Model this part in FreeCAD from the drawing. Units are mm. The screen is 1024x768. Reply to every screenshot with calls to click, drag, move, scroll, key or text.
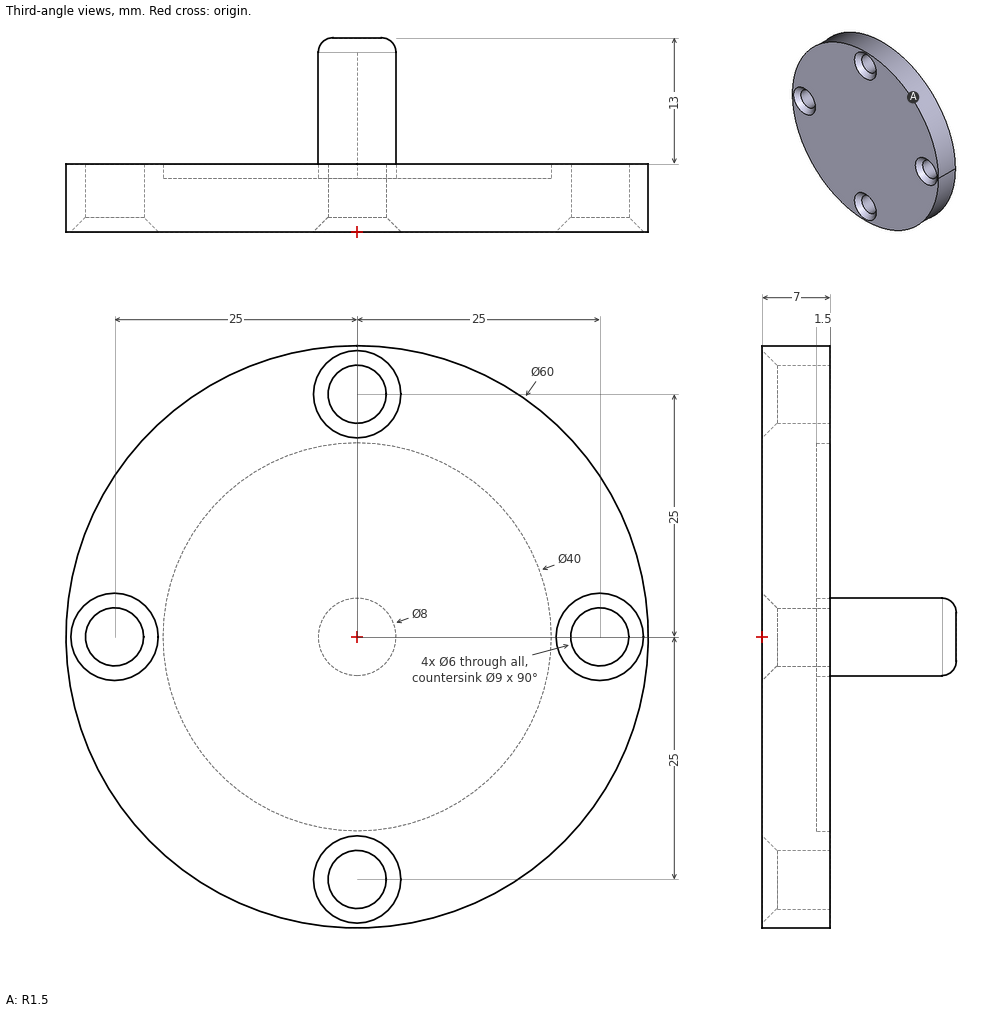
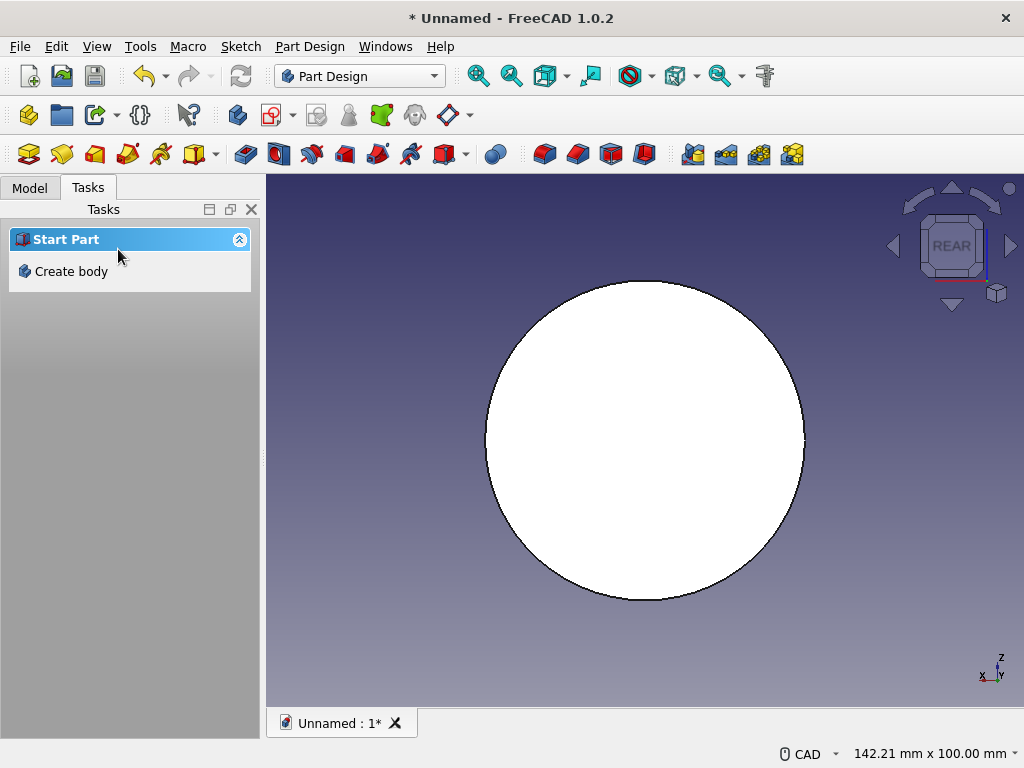
click(645, 439)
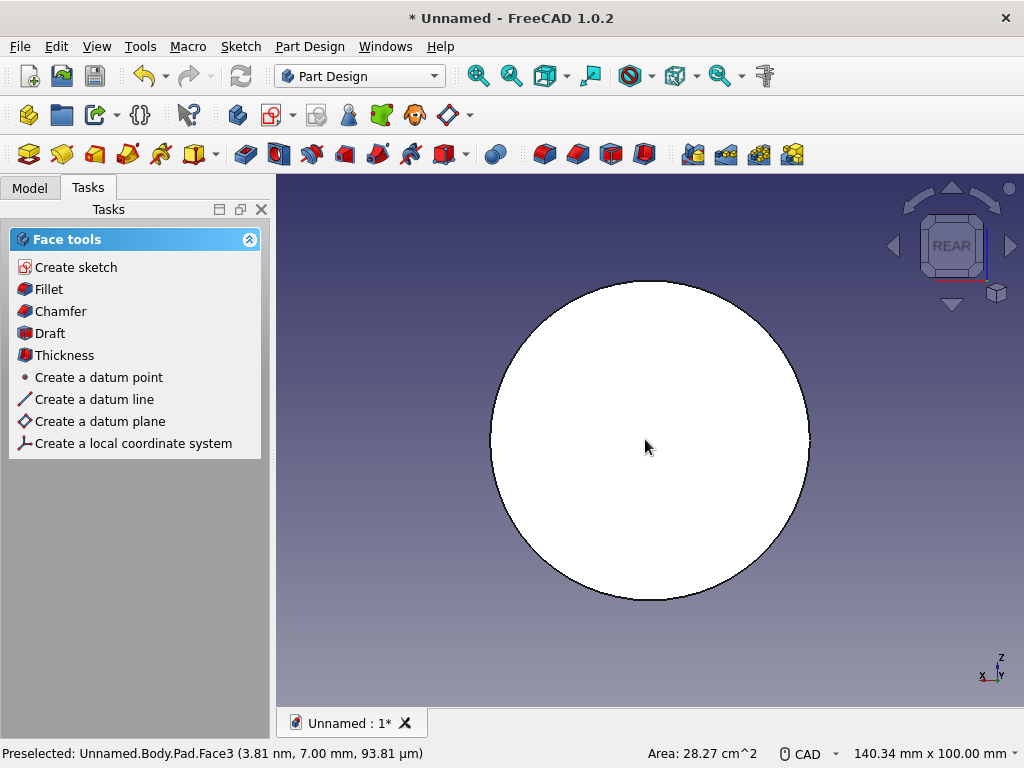
click(270, 116)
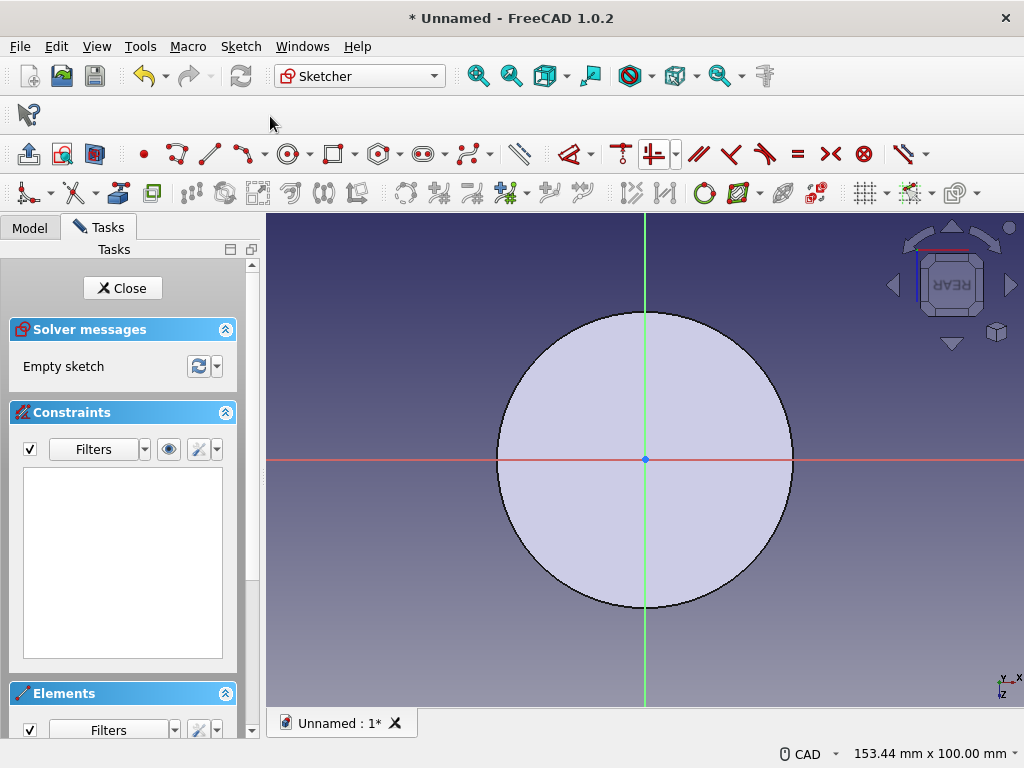
scroll(656, 460, up, 10)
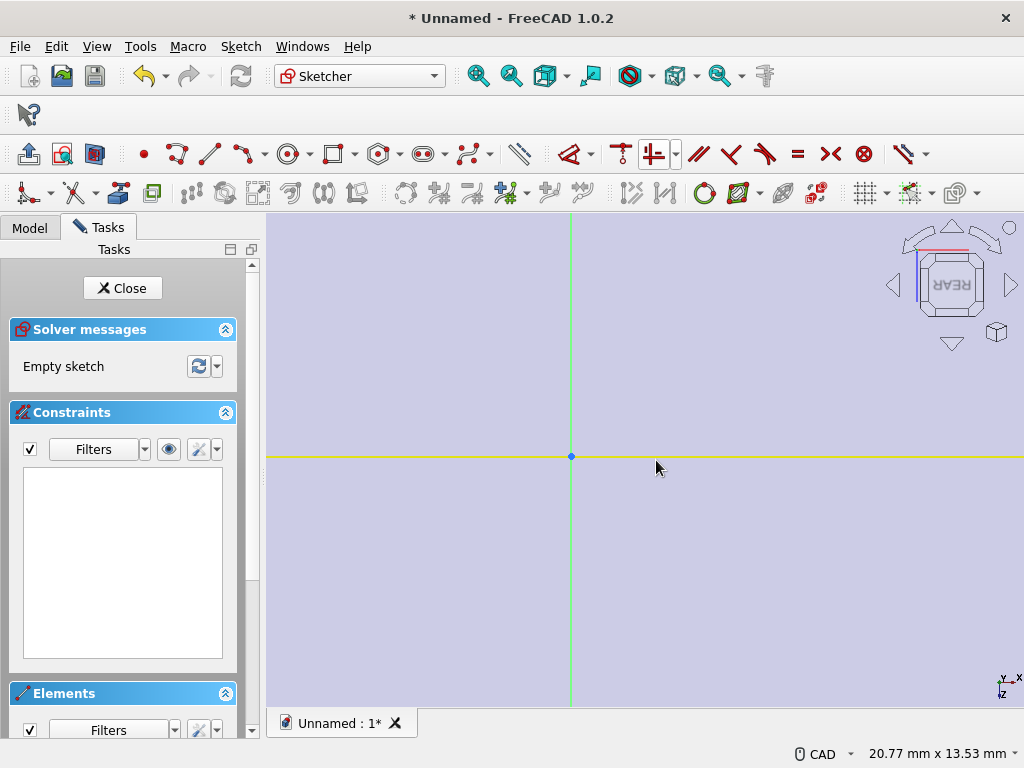
click(288, 154)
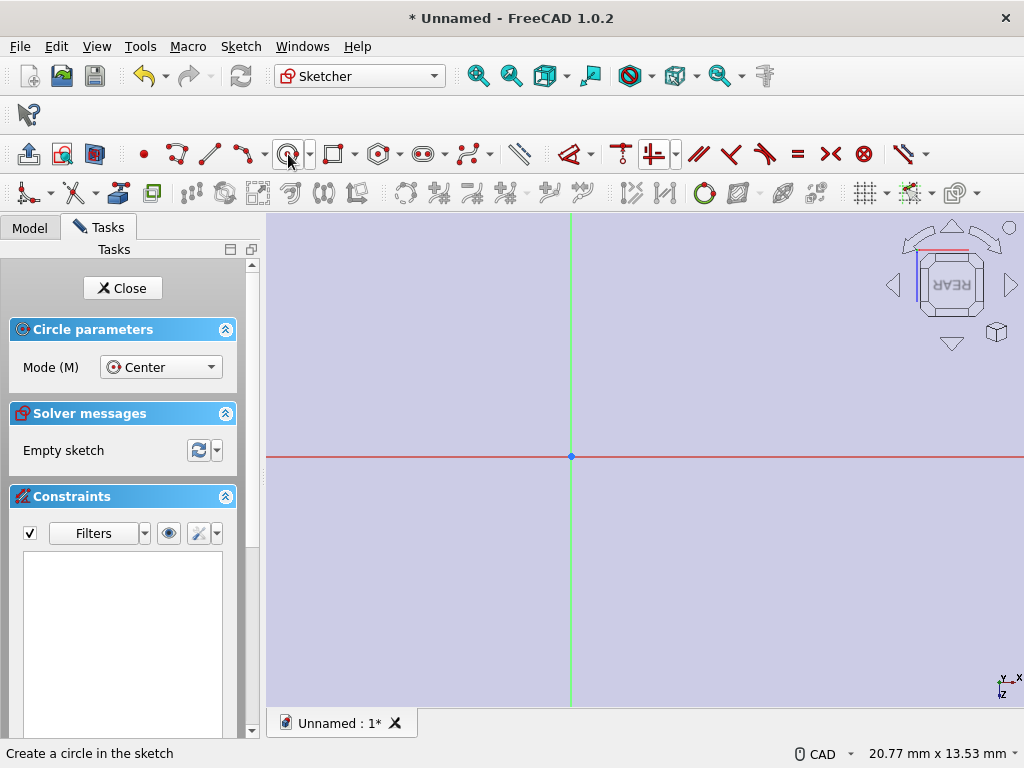
click(571, 457)
move(675, 354)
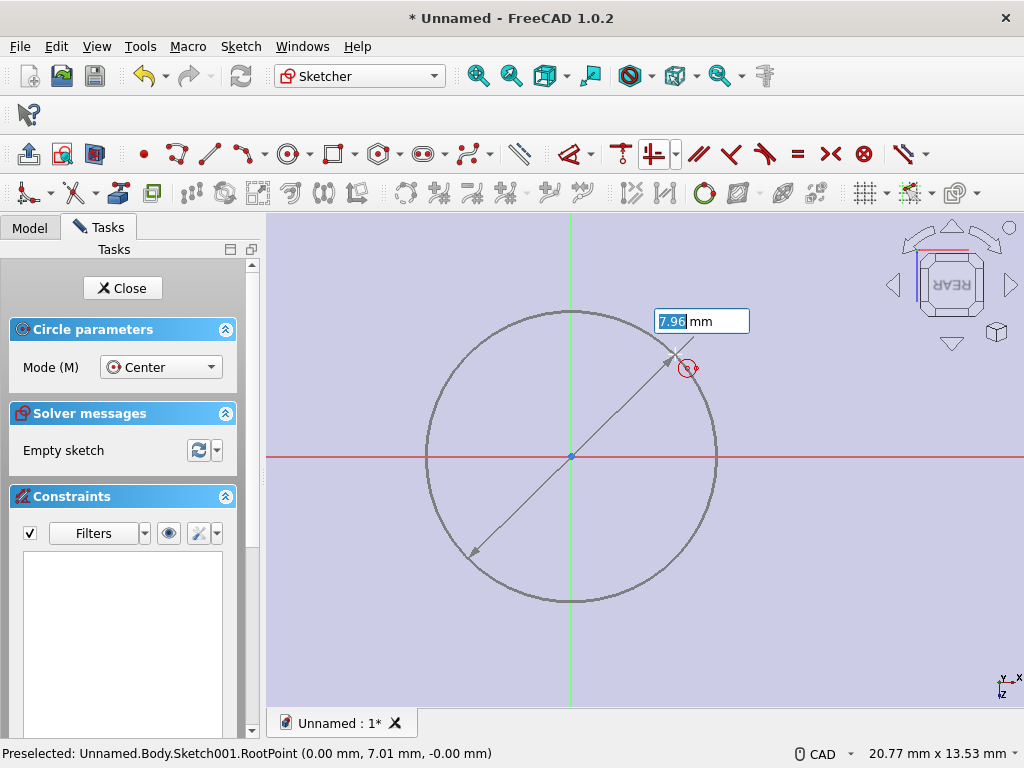
text(8)
key(Return)
key(Escape)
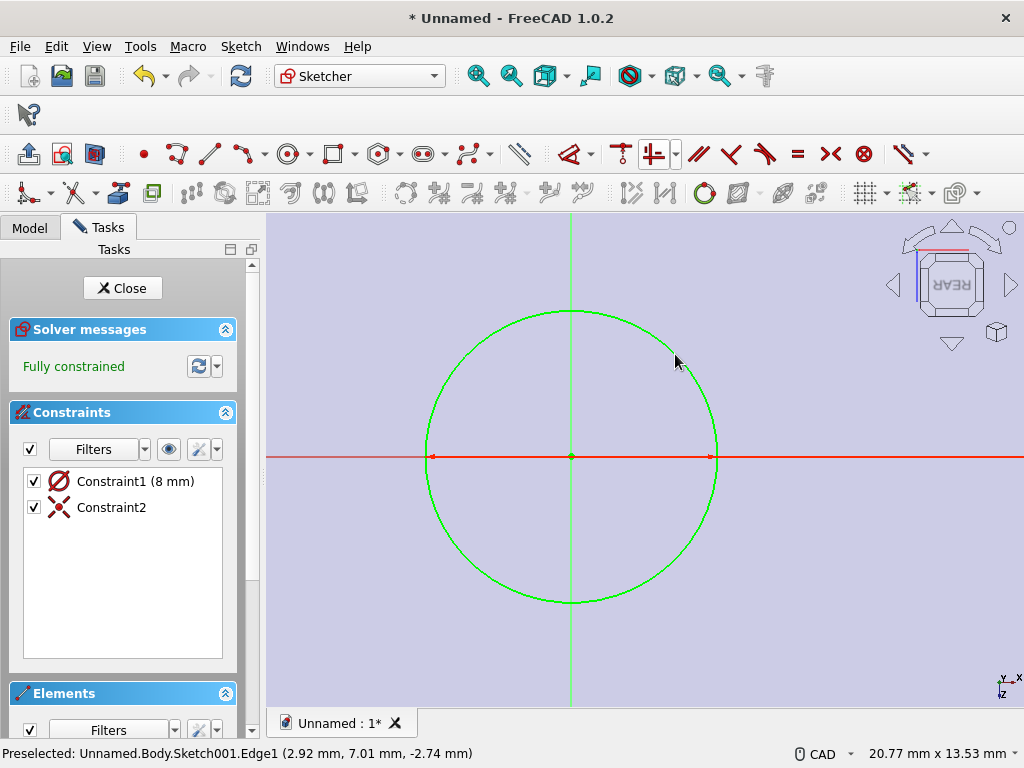
click(123, 288)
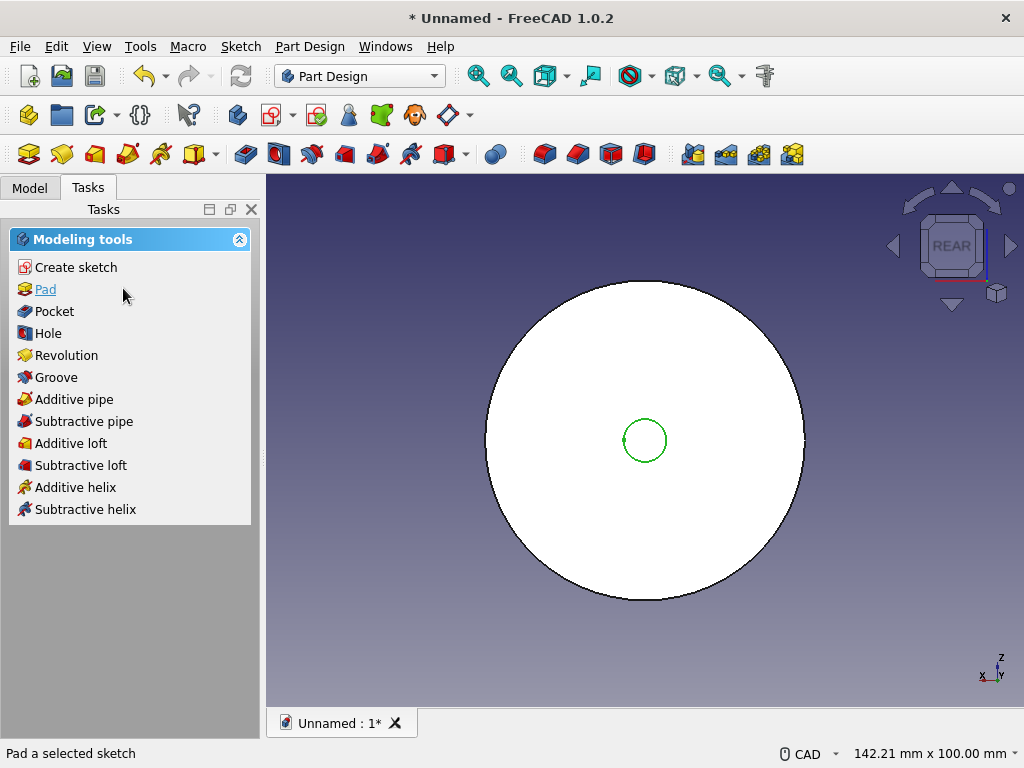
click(29, 154)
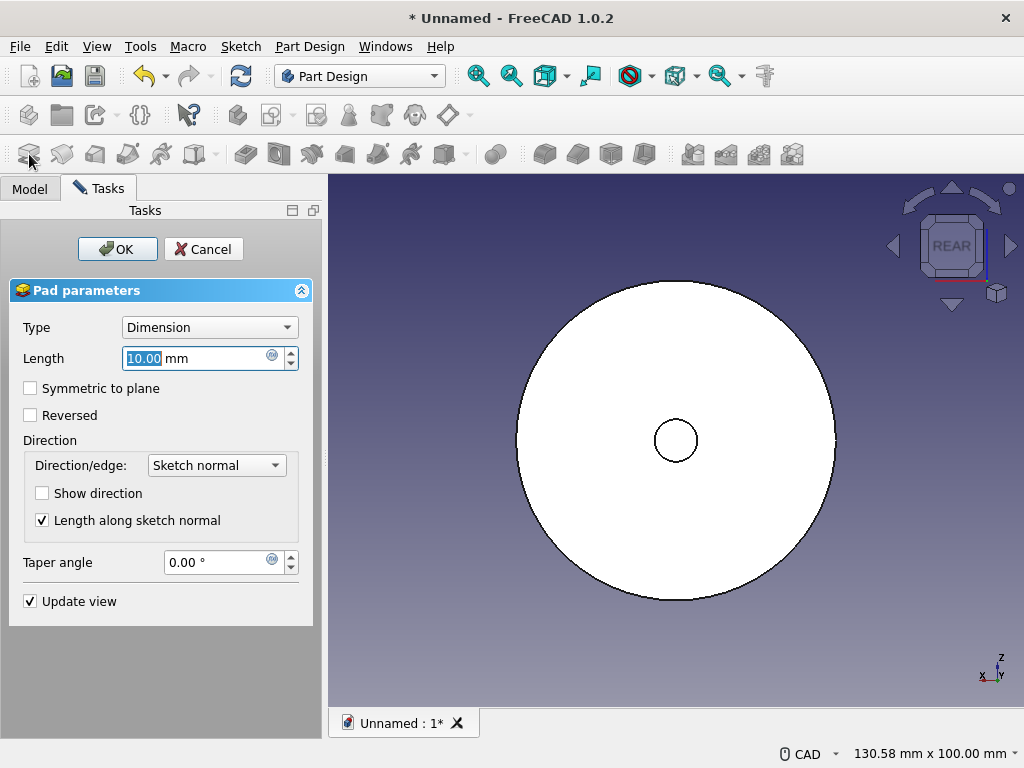
text(13)
key(Tab)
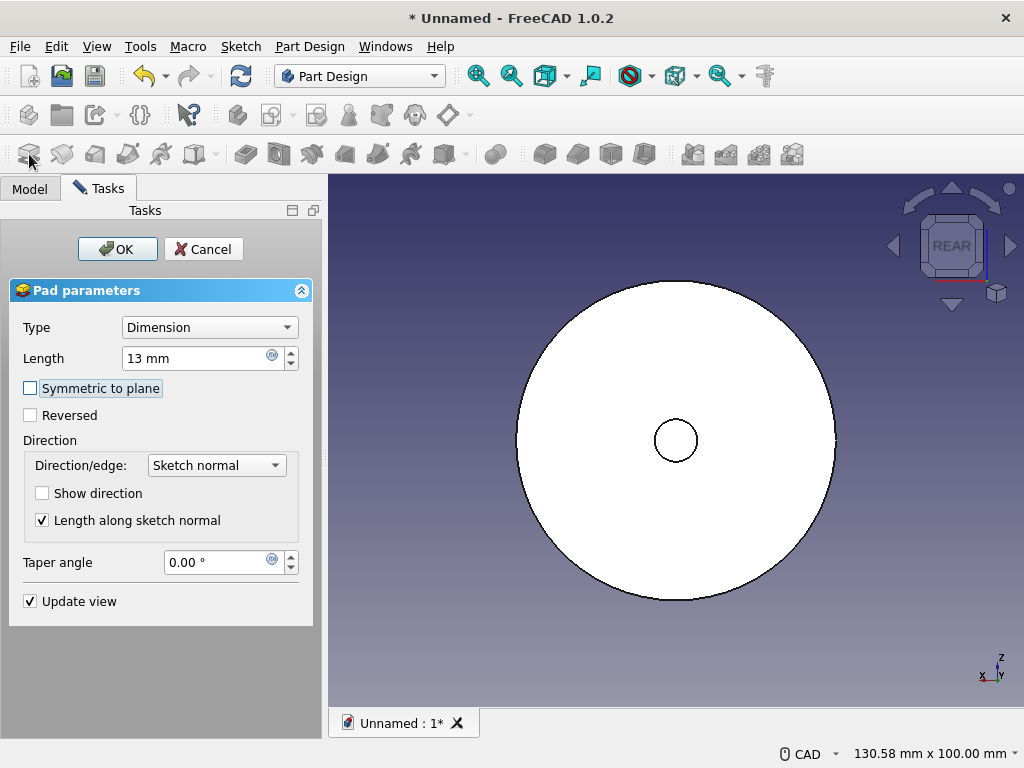
click(118, 249)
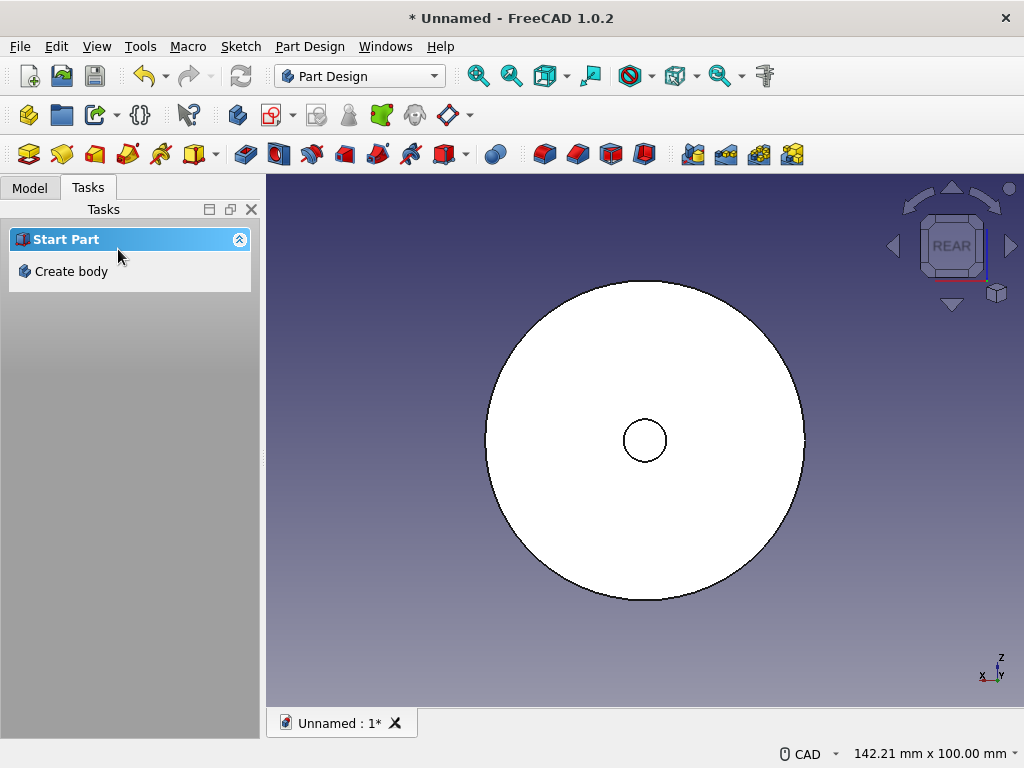
click(30, 188)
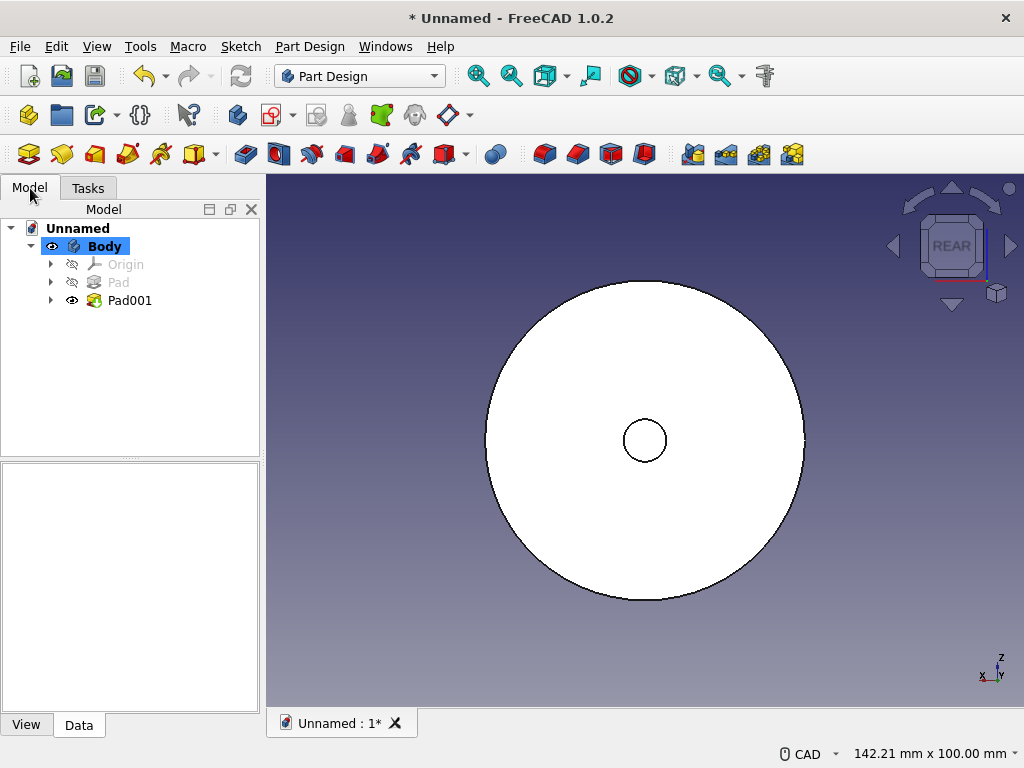
click(51, 264)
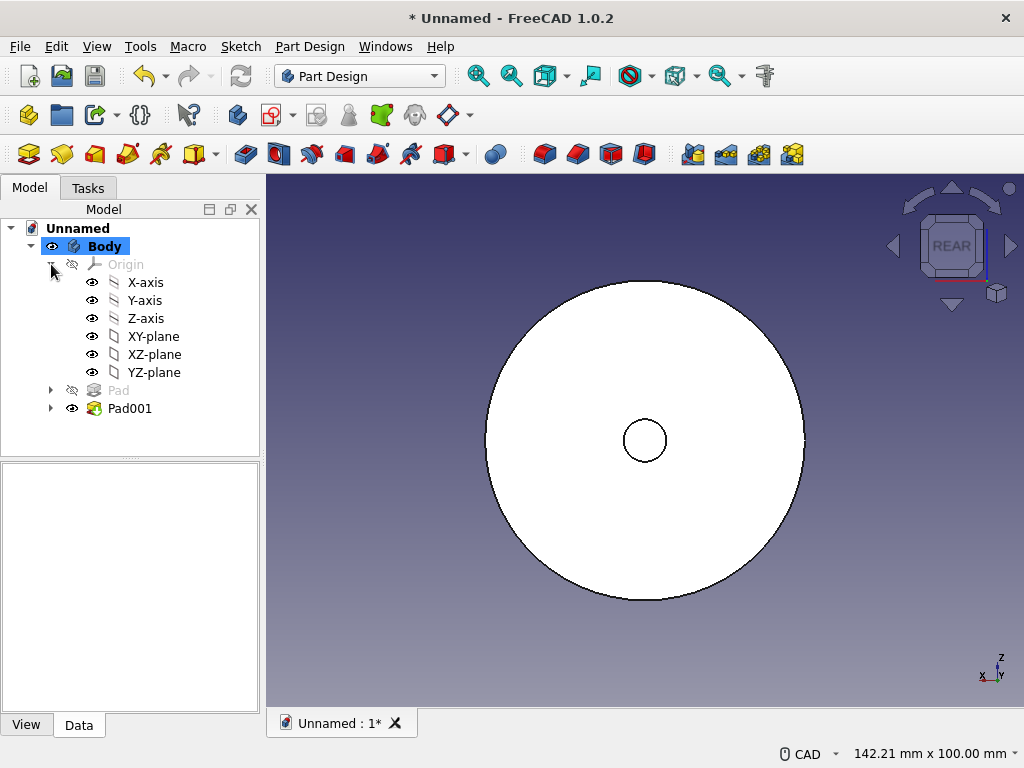
click(137, 354)